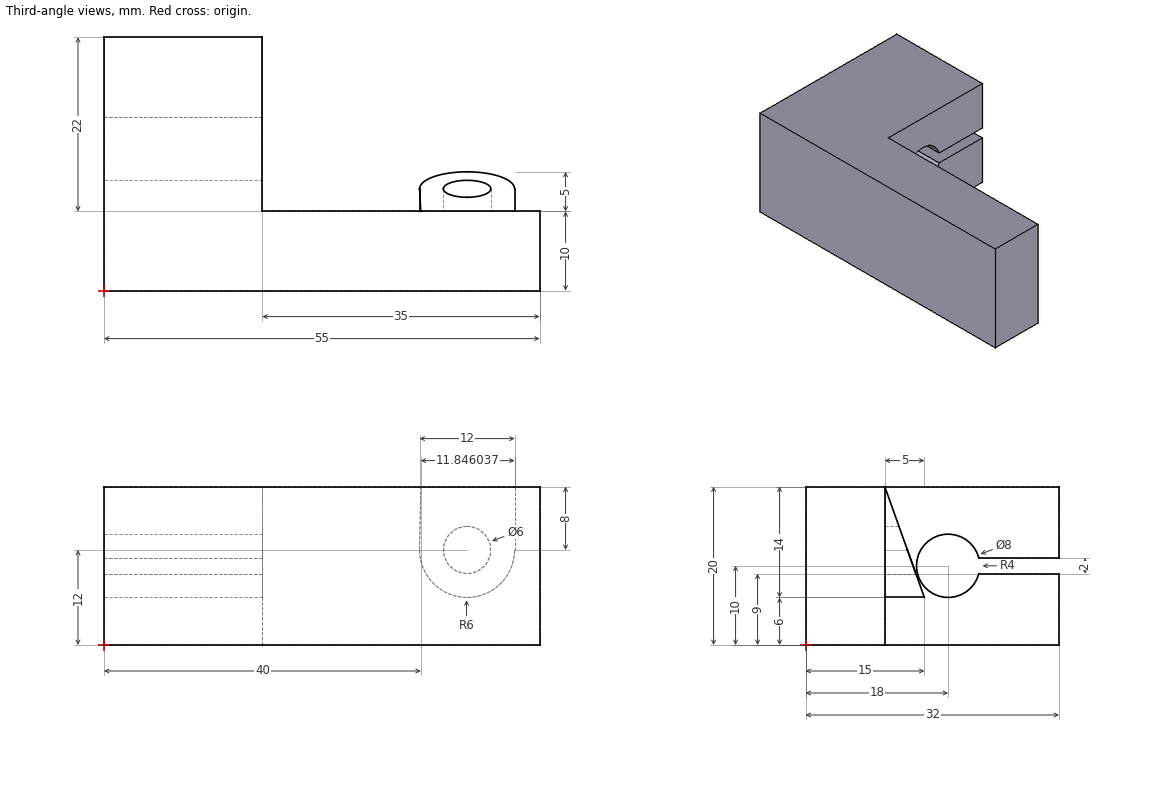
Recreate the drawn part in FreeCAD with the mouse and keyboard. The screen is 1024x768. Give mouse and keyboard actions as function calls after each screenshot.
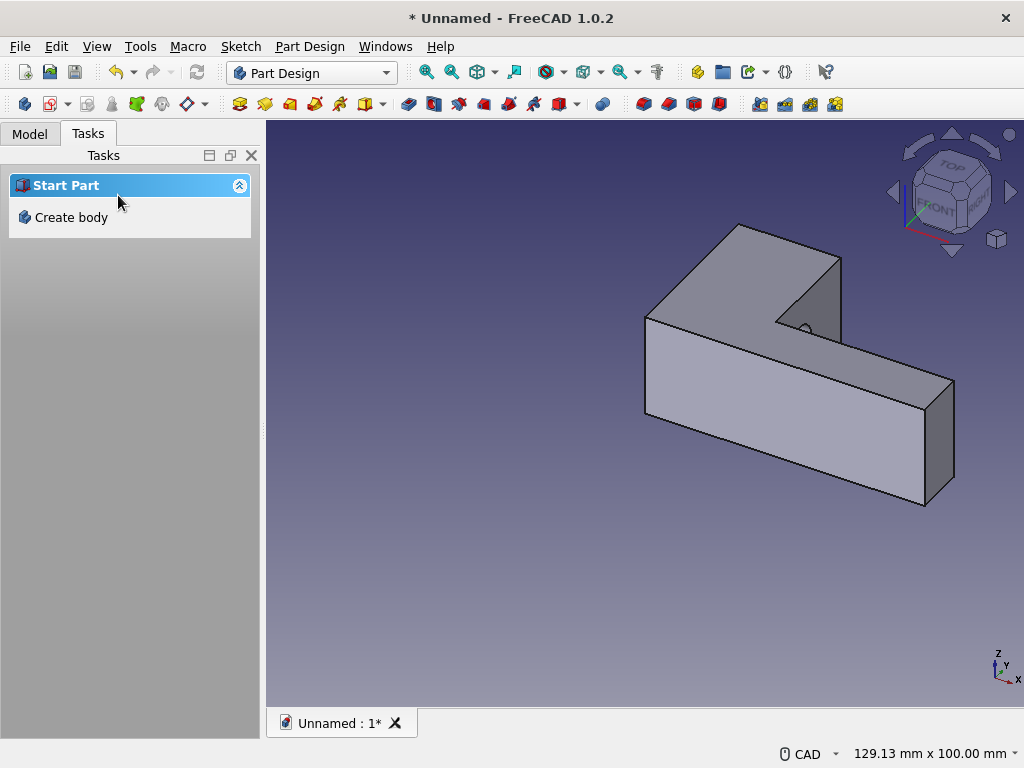
click(827, 305)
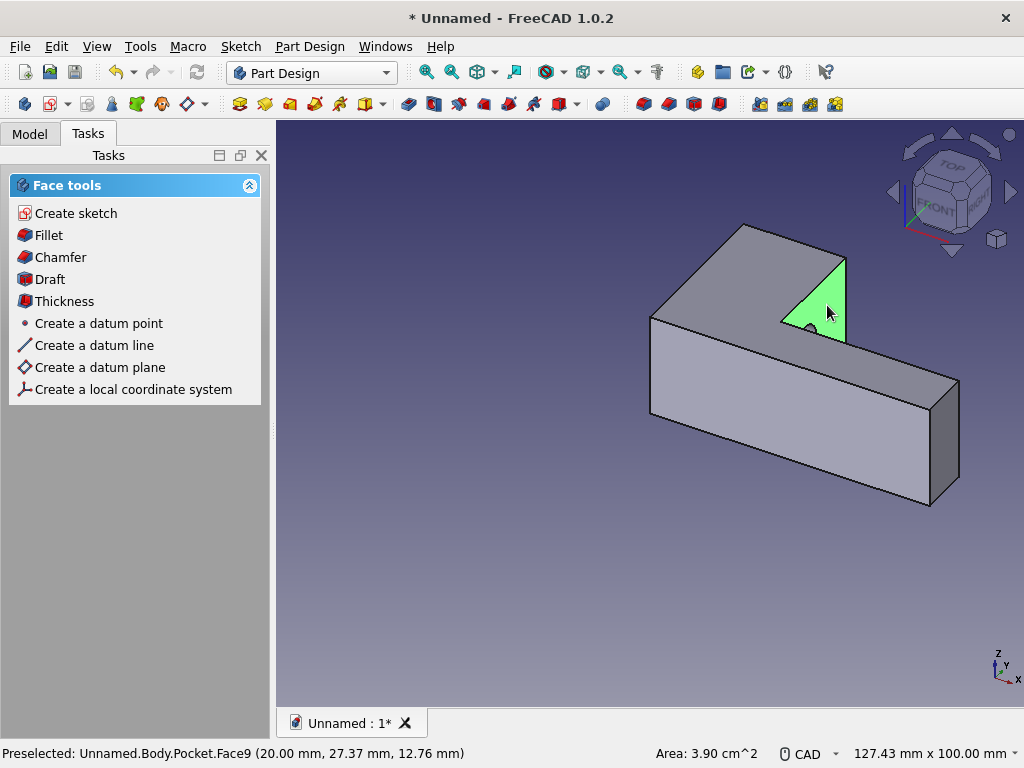
click(50, 104)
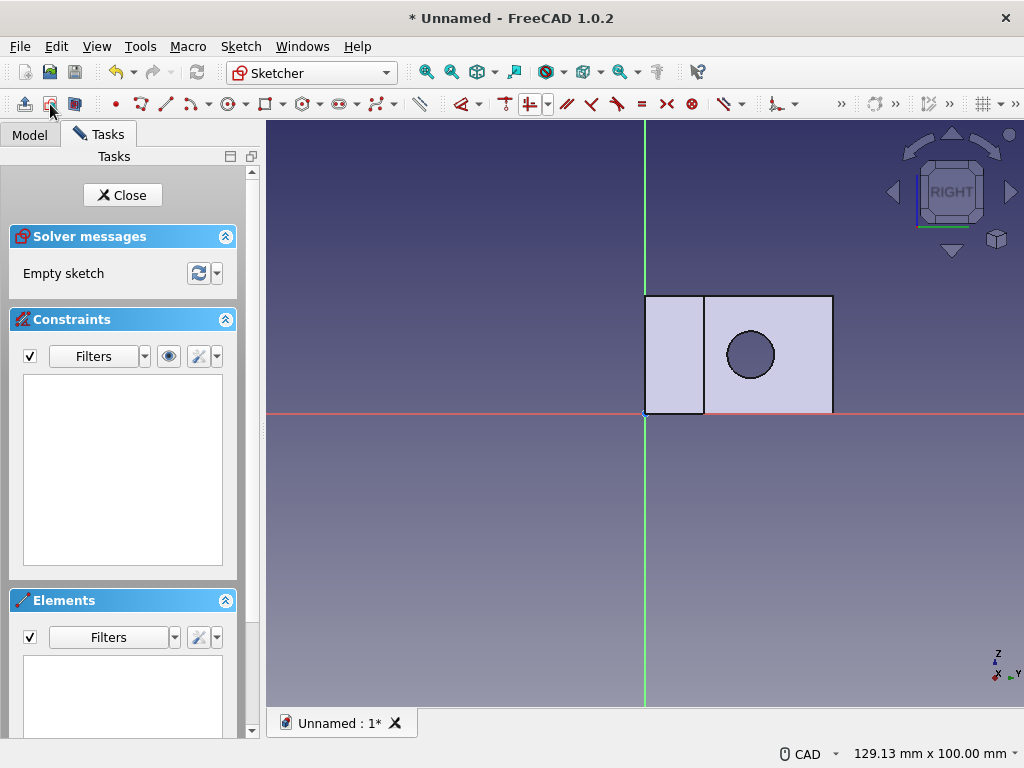
key(q)
key(s)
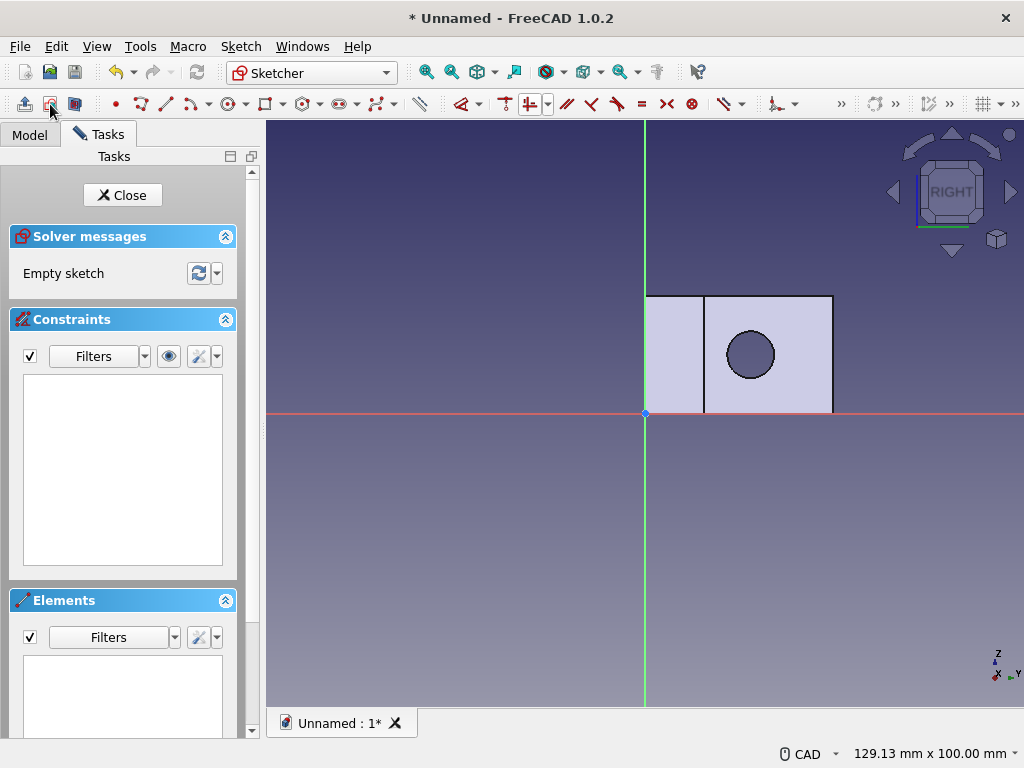
scroll(839, 346, up, 10)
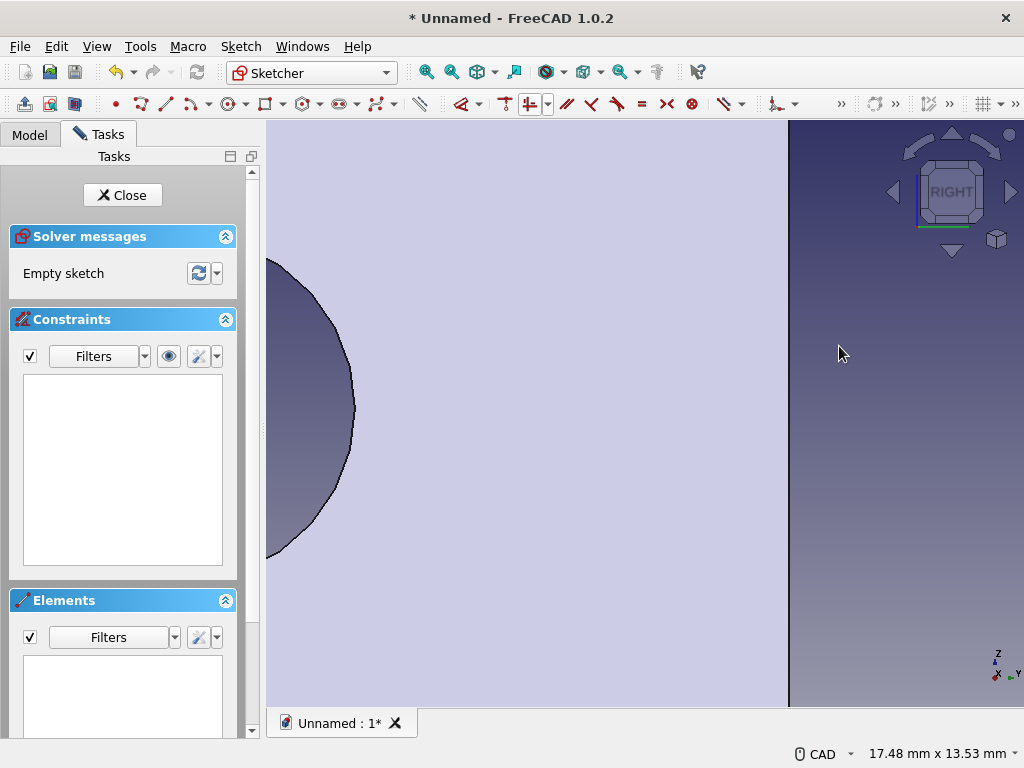
click(141, 104)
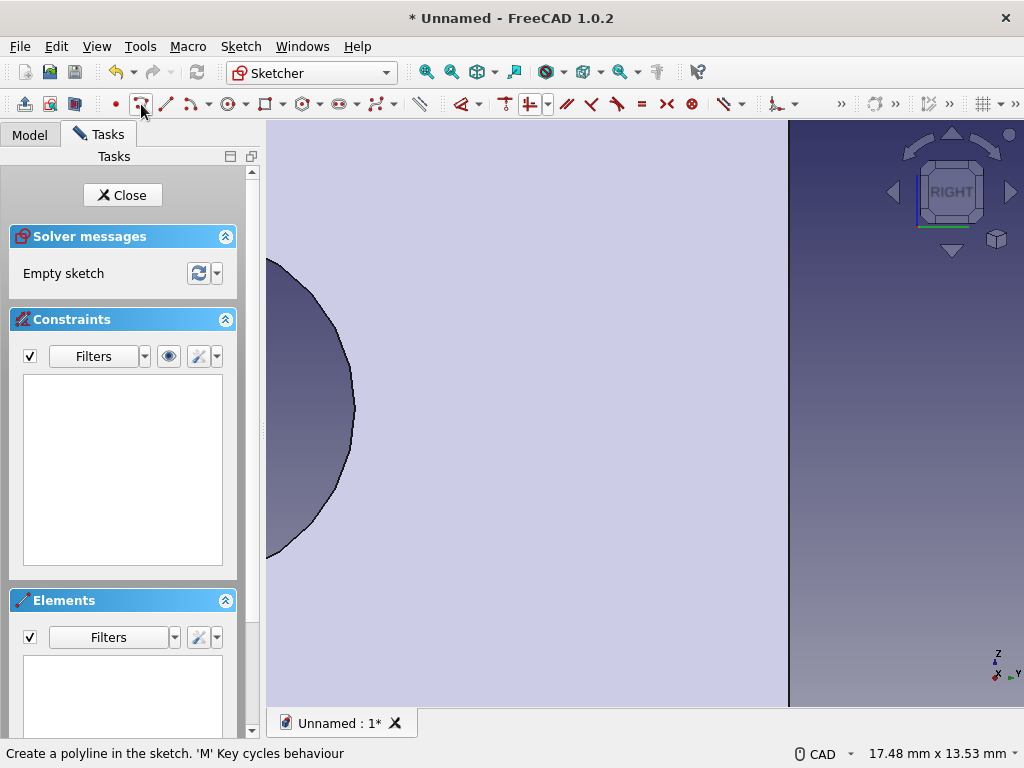
click(349, 452)
click(789, 452)
click(789, 365)
click(349, 365)
right_click(349, 365)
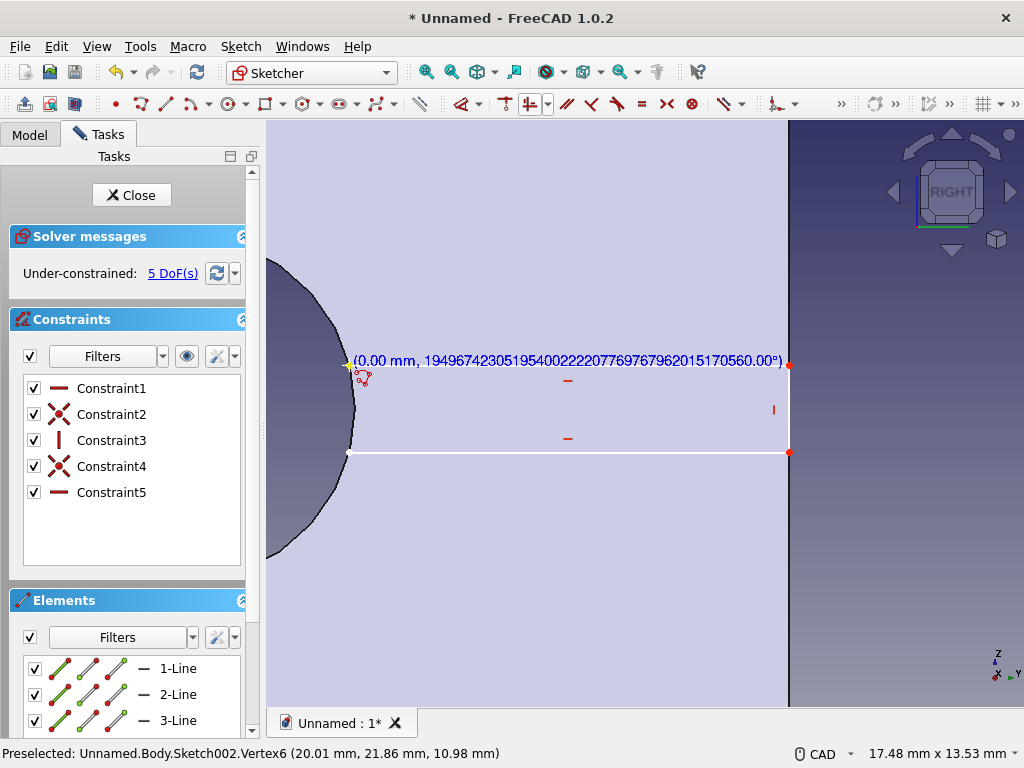
key(g)
key(3)
key(a)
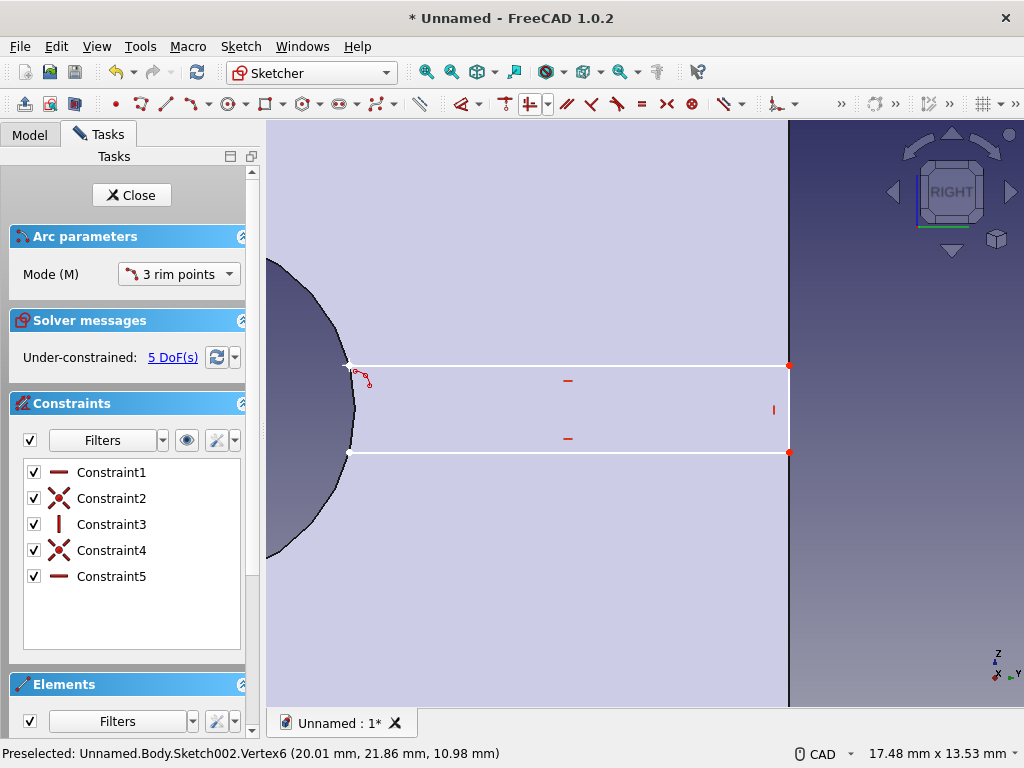
click(349, 366)
click(349, 453)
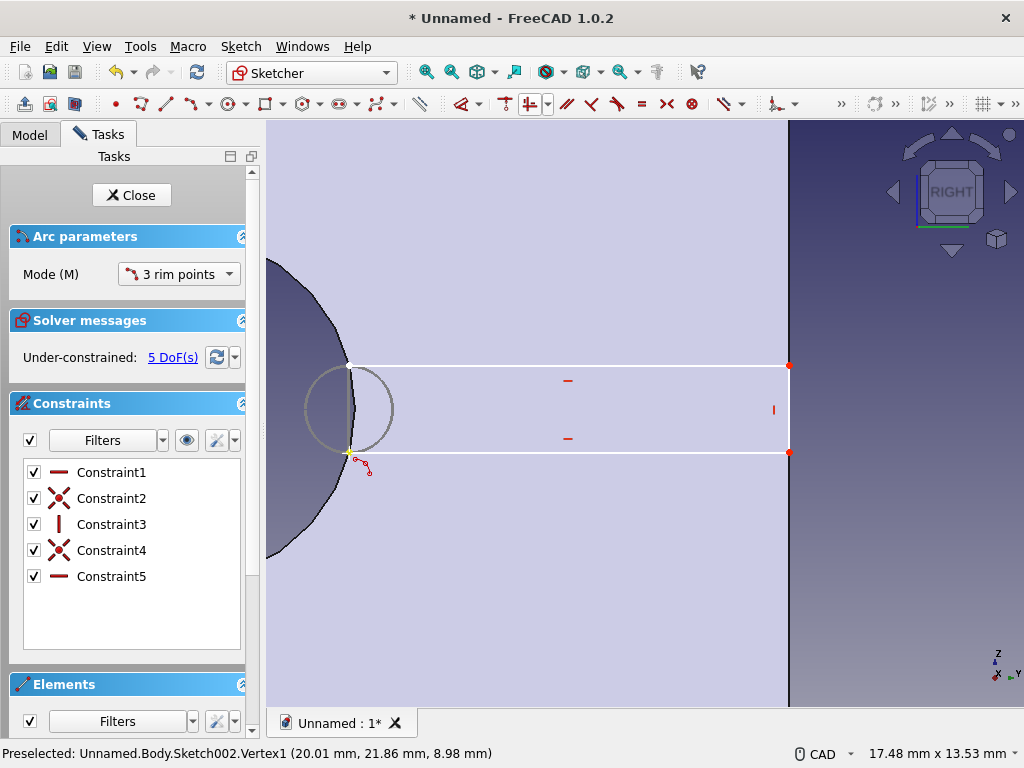
scroll(355, 409, up, 6)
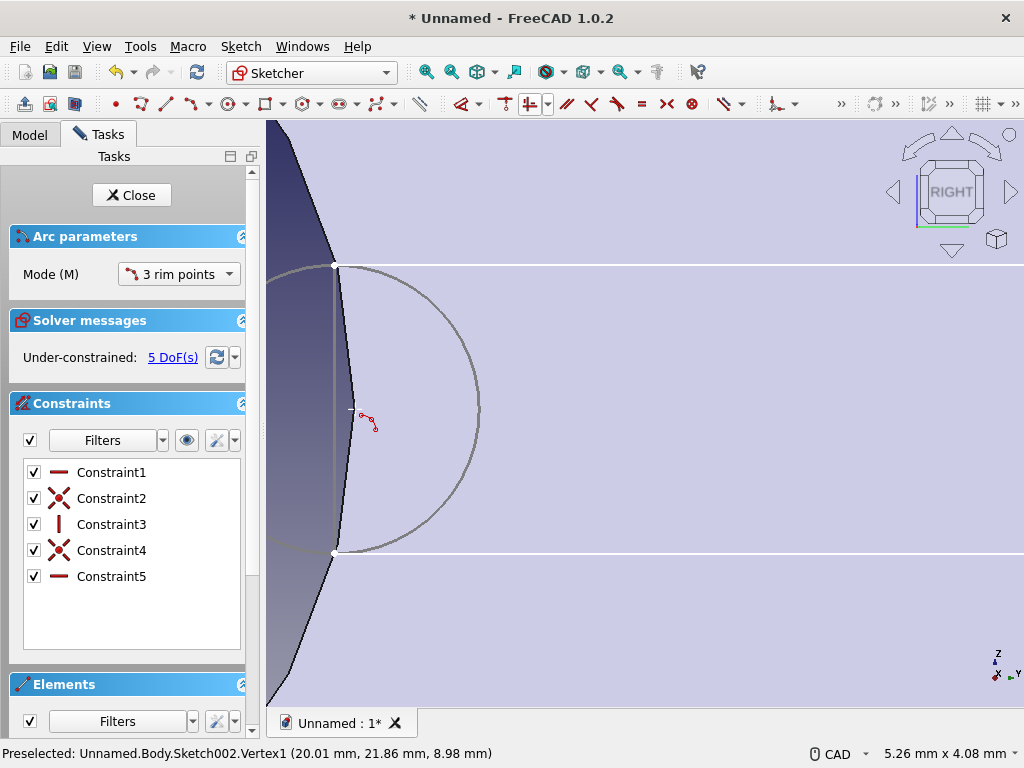
click(354, 406)
key(Escape)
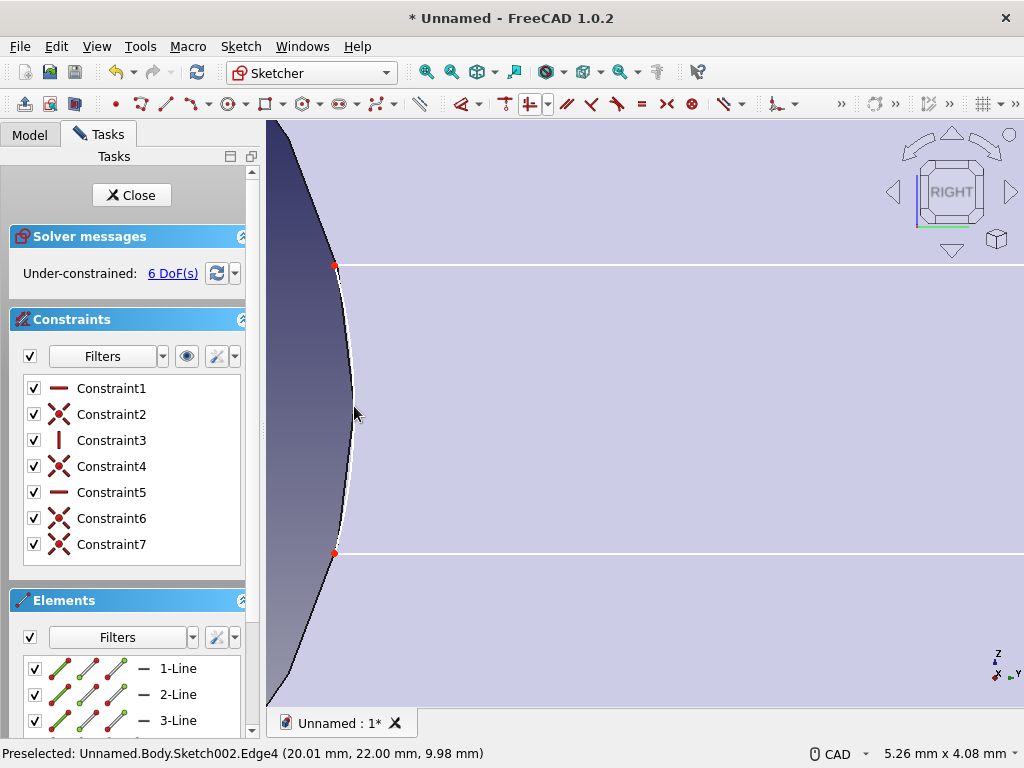
click(460, 104)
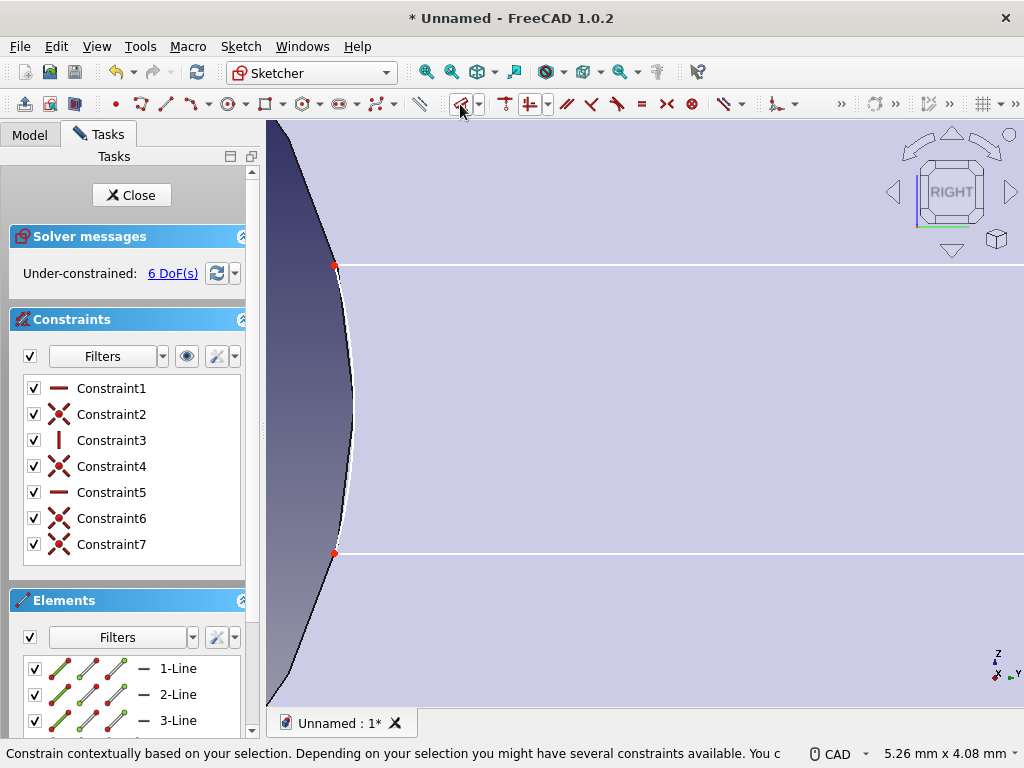
click(351, 468)
click(383, 471)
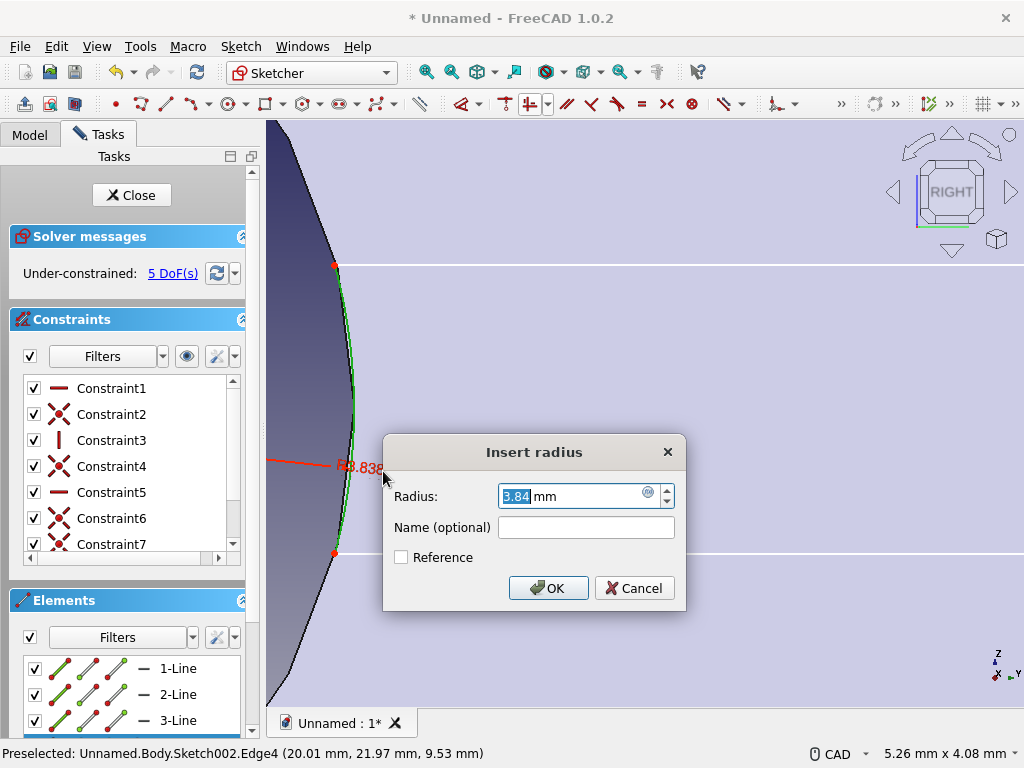
text(4)
key(Return)